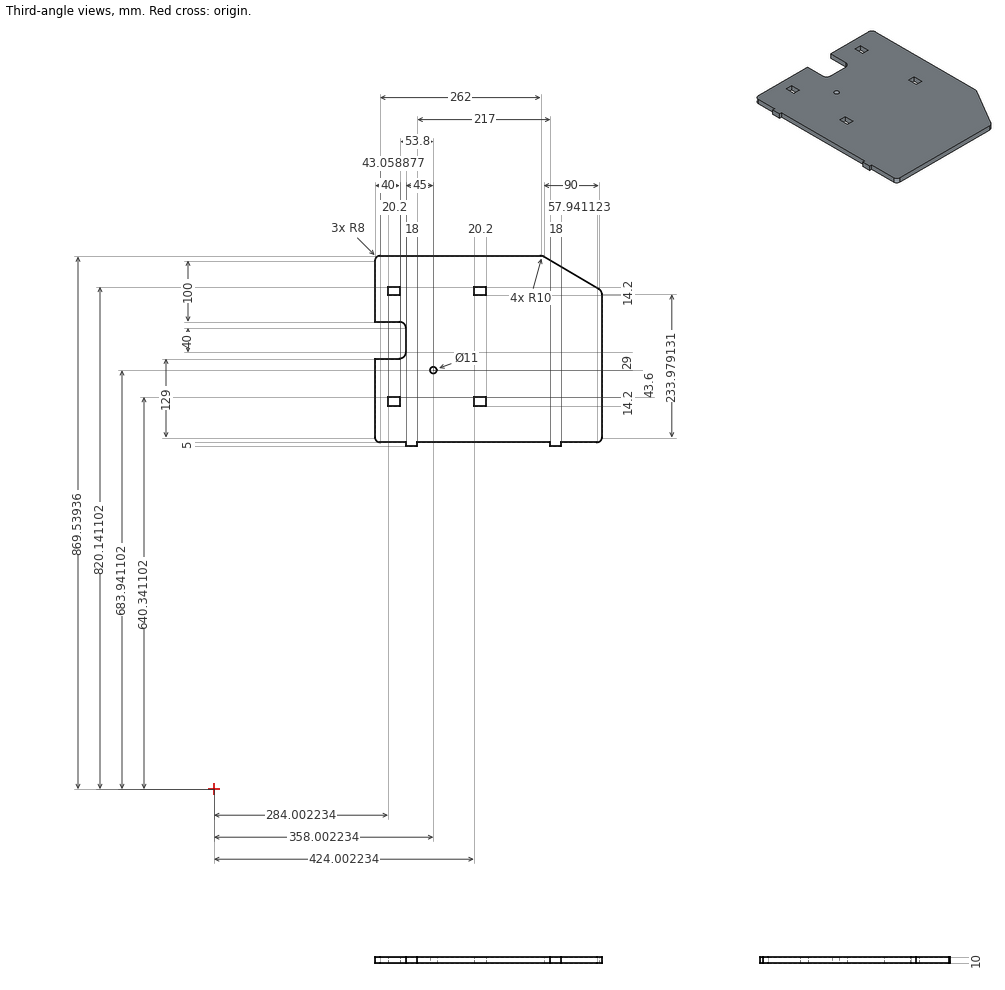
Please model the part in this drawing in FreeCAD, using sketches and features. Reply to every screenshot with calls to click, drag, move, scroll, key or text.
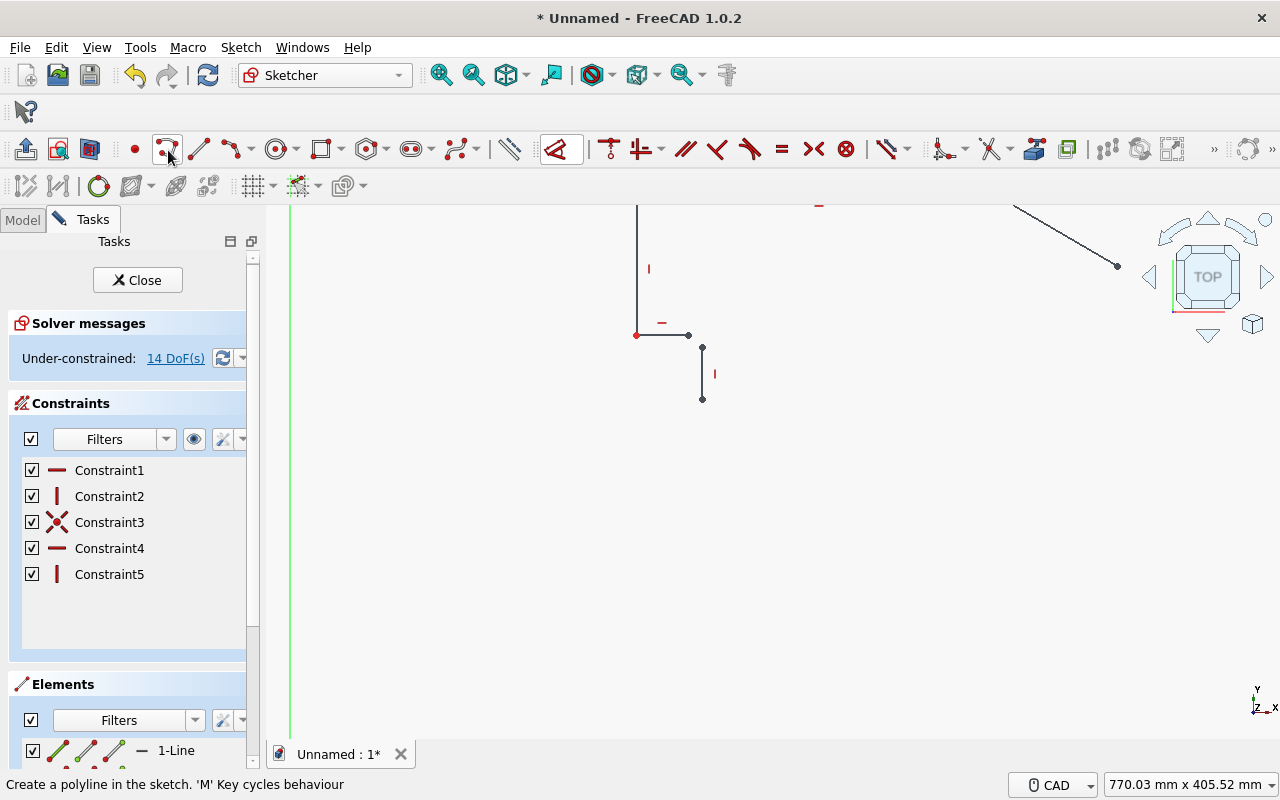
click(689, 412)
click(637, 412)
click(637, 582)
right_click(637, 582)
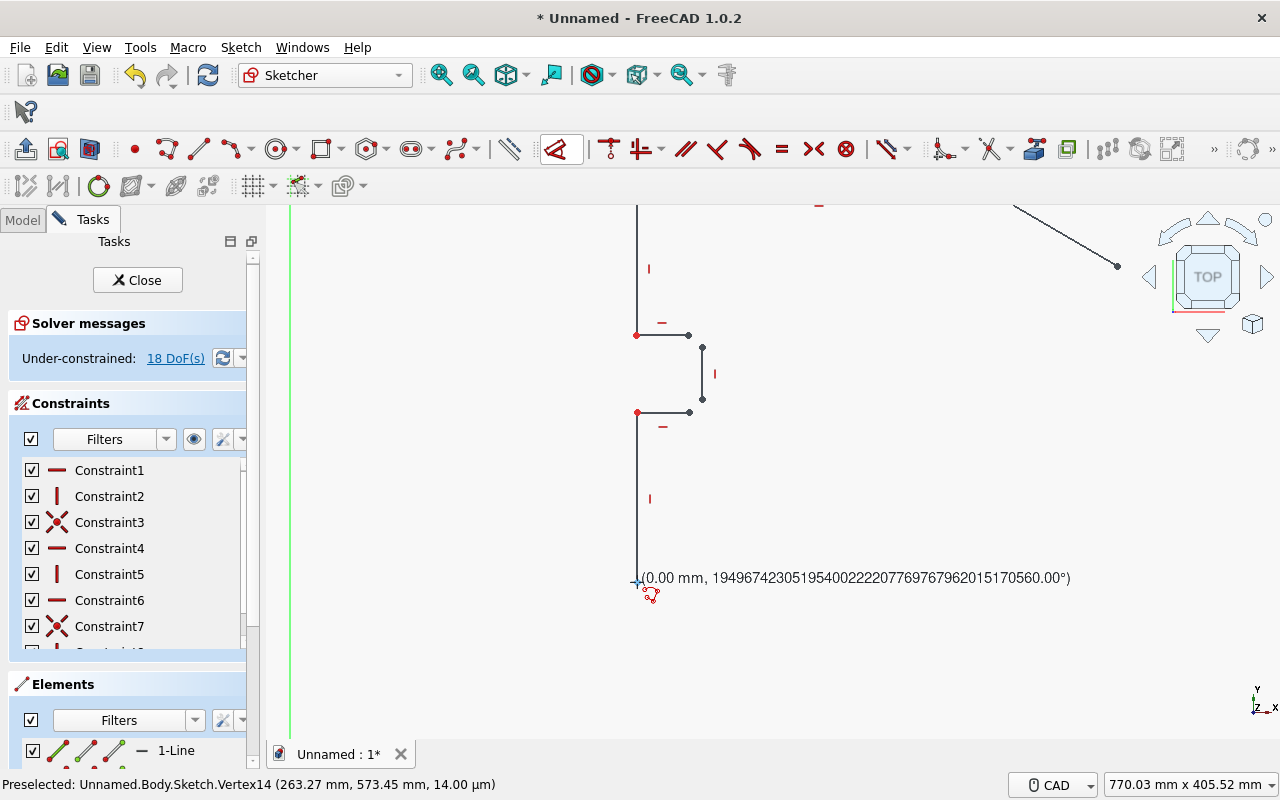
click(647, 593)
click(704, 593)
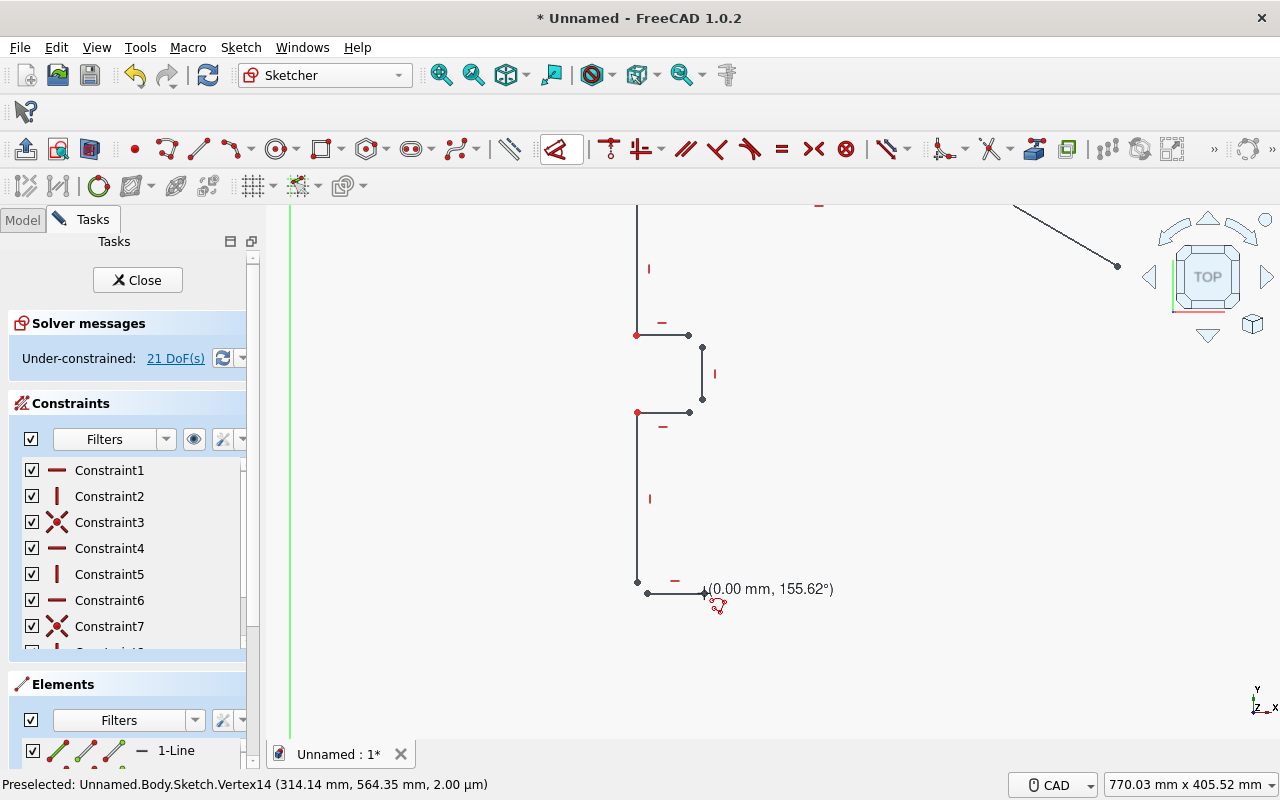
scroll(704, 599, up, 5)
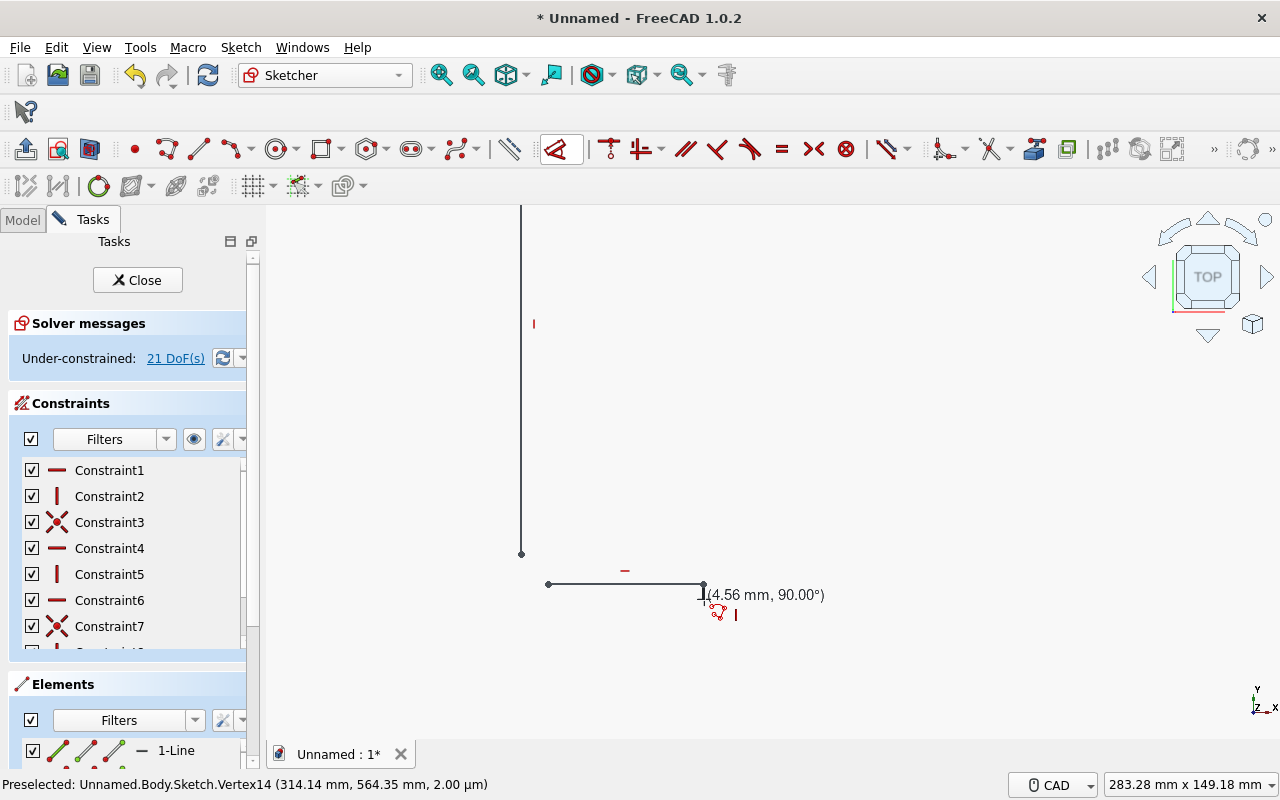
click(703, 599)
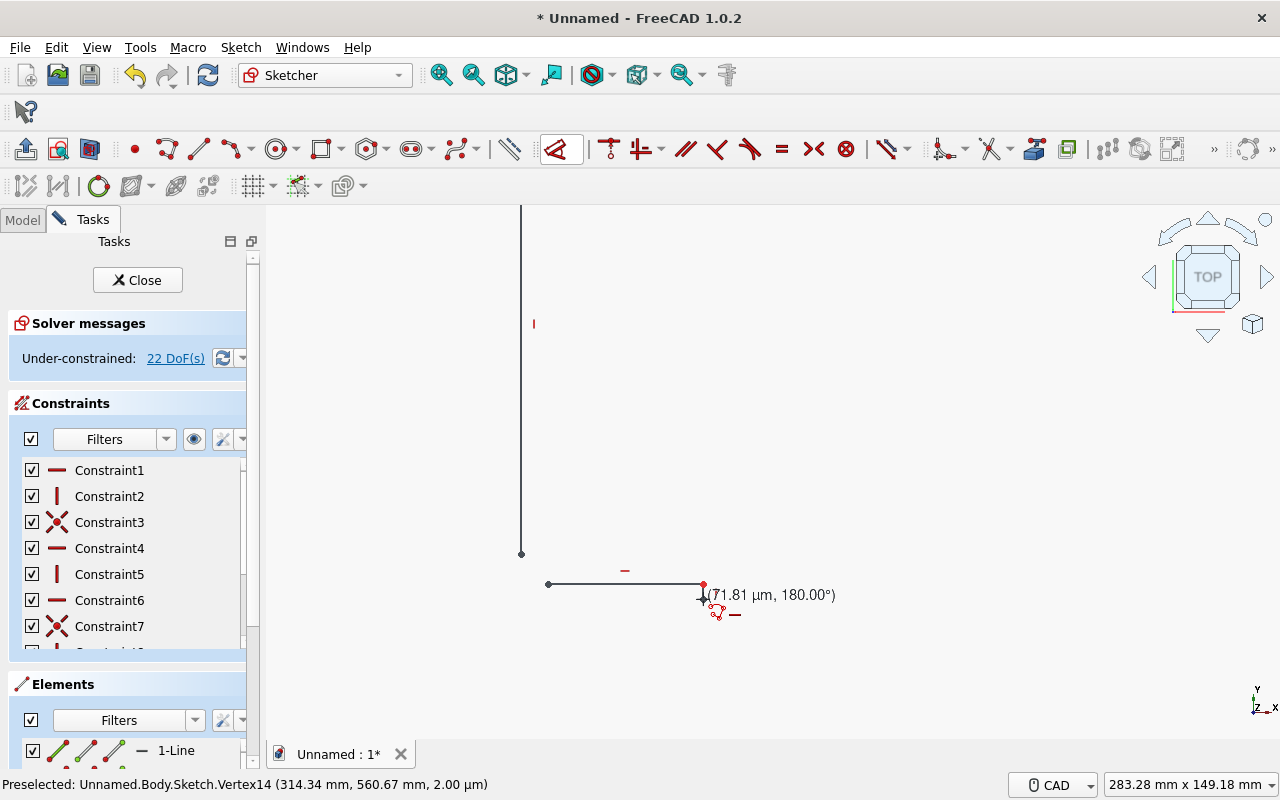
scroll(704, 400, down, 11)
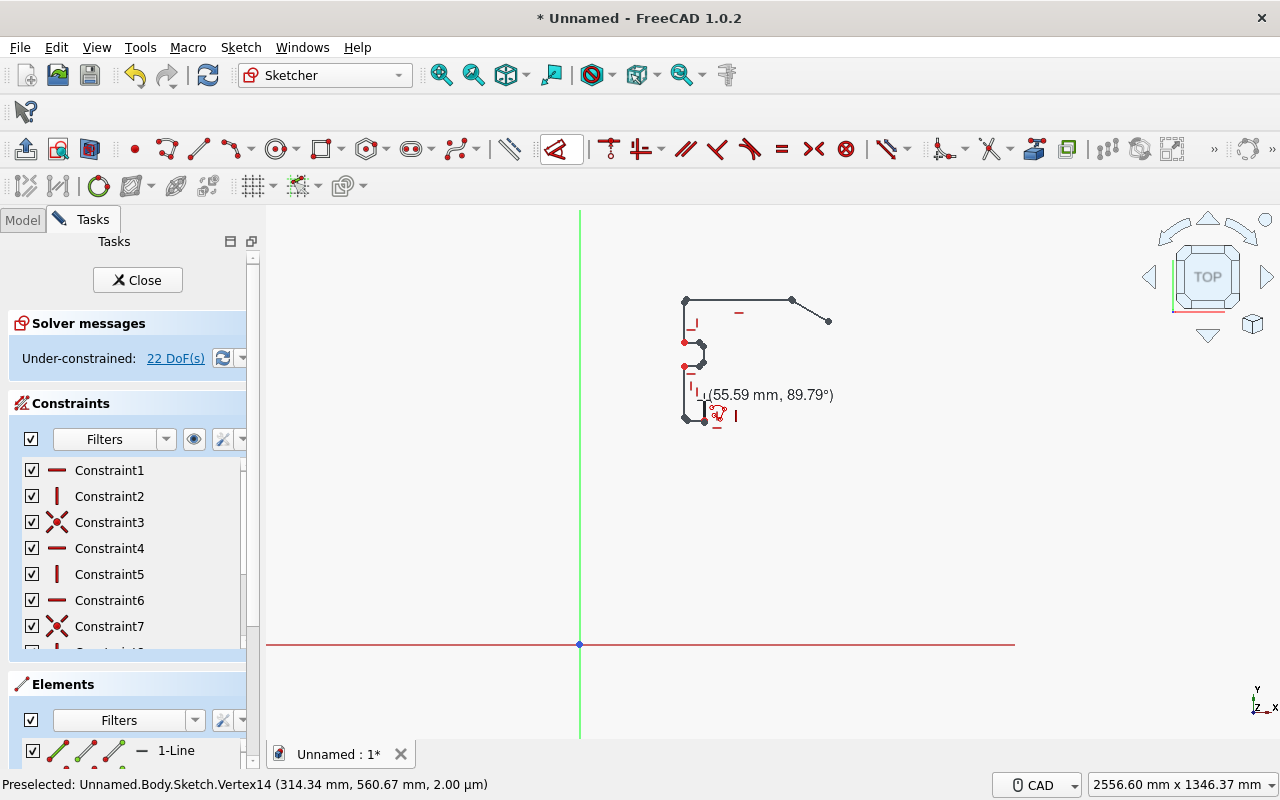
scroll(711, 422, up, 4)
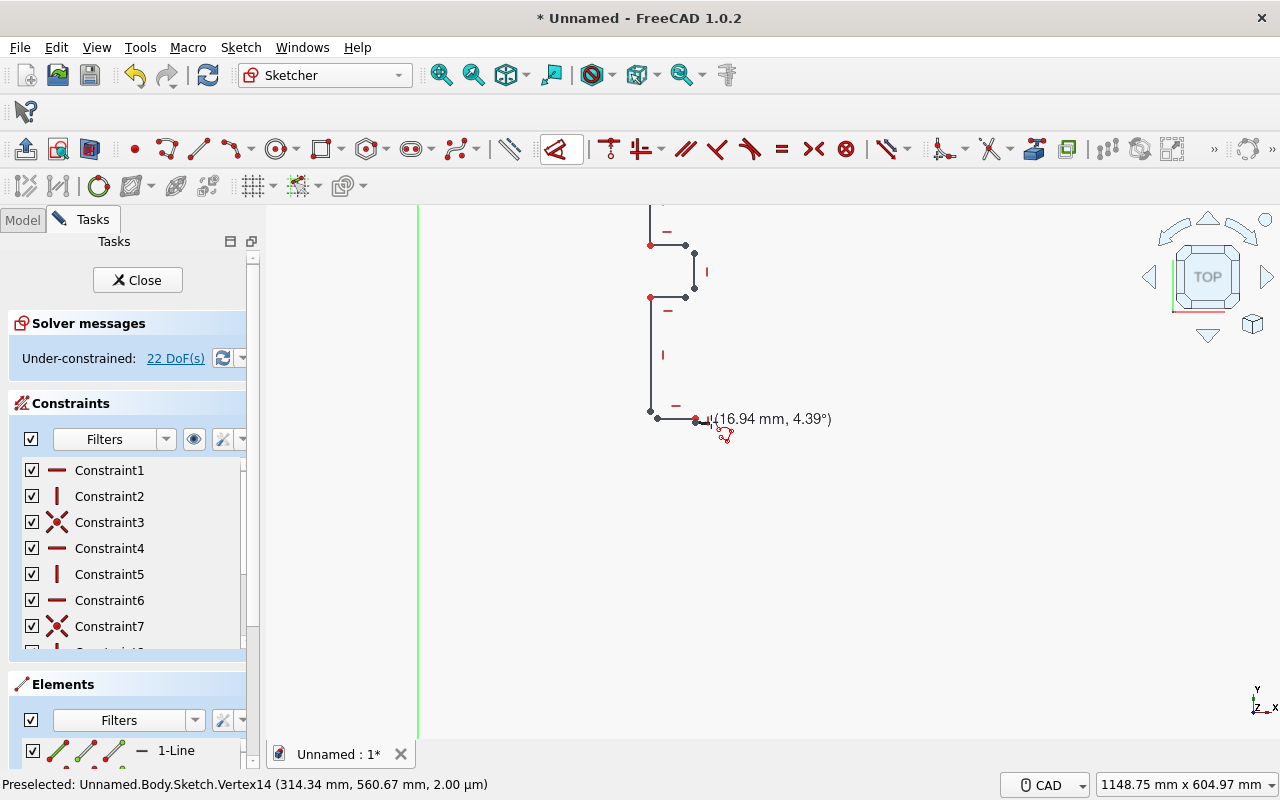
click(711, 422)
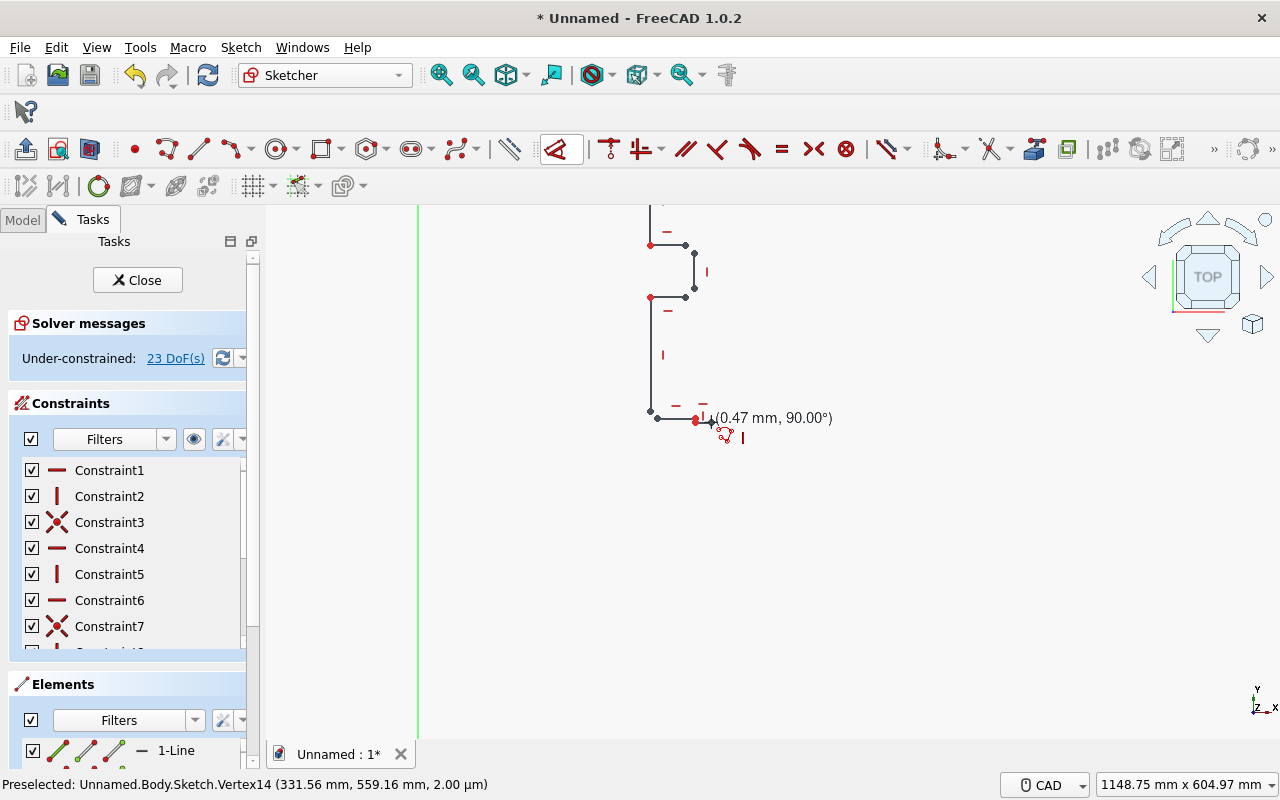
scroll(711, 418, up, 7)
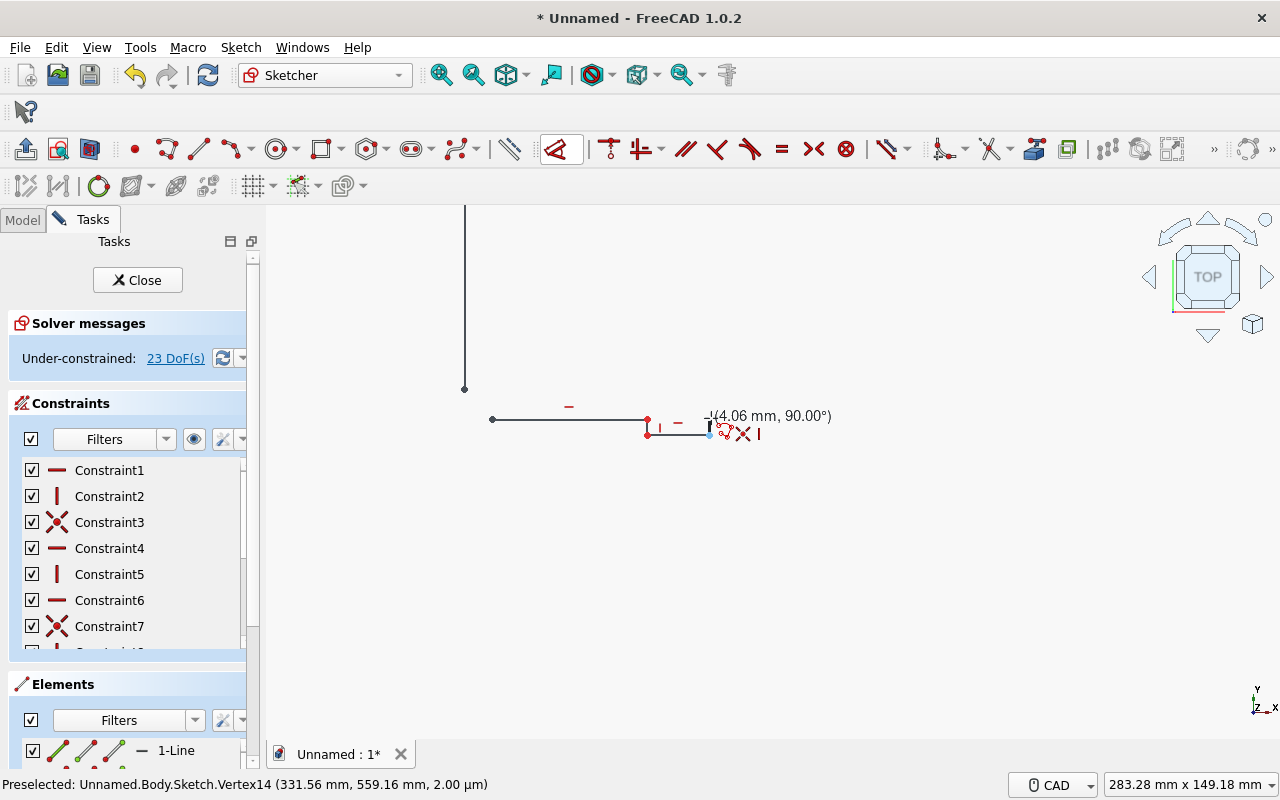
click(710, 416)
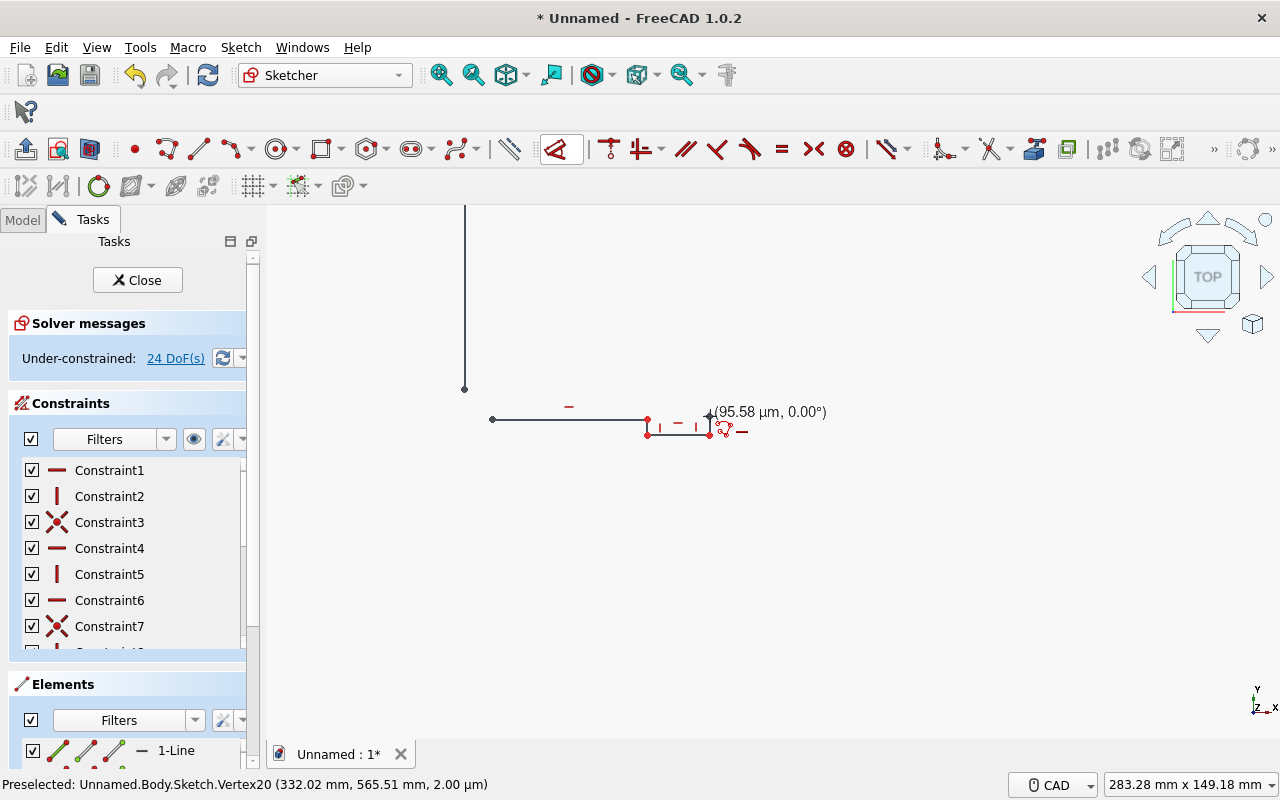
scroll(711, 421, down, 11)